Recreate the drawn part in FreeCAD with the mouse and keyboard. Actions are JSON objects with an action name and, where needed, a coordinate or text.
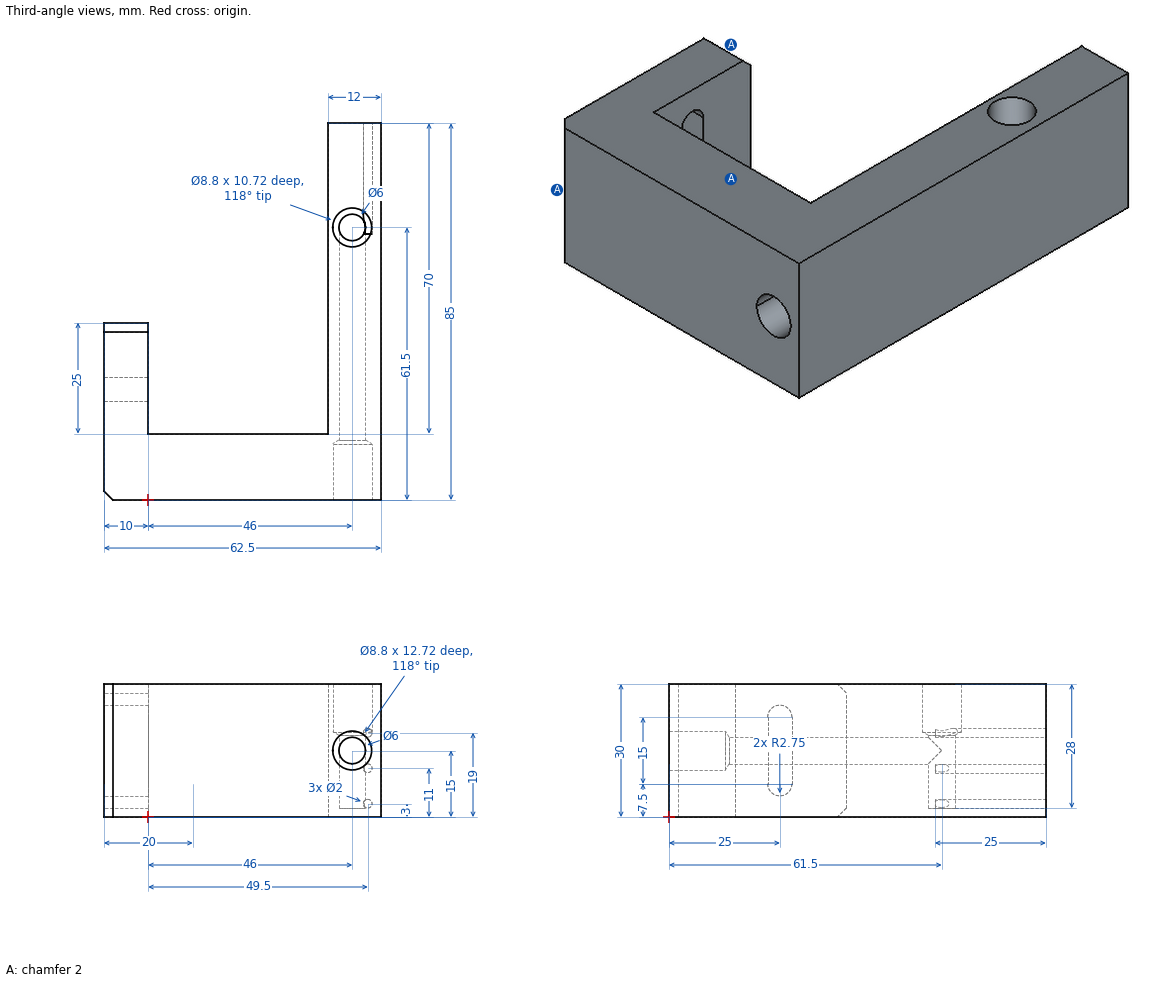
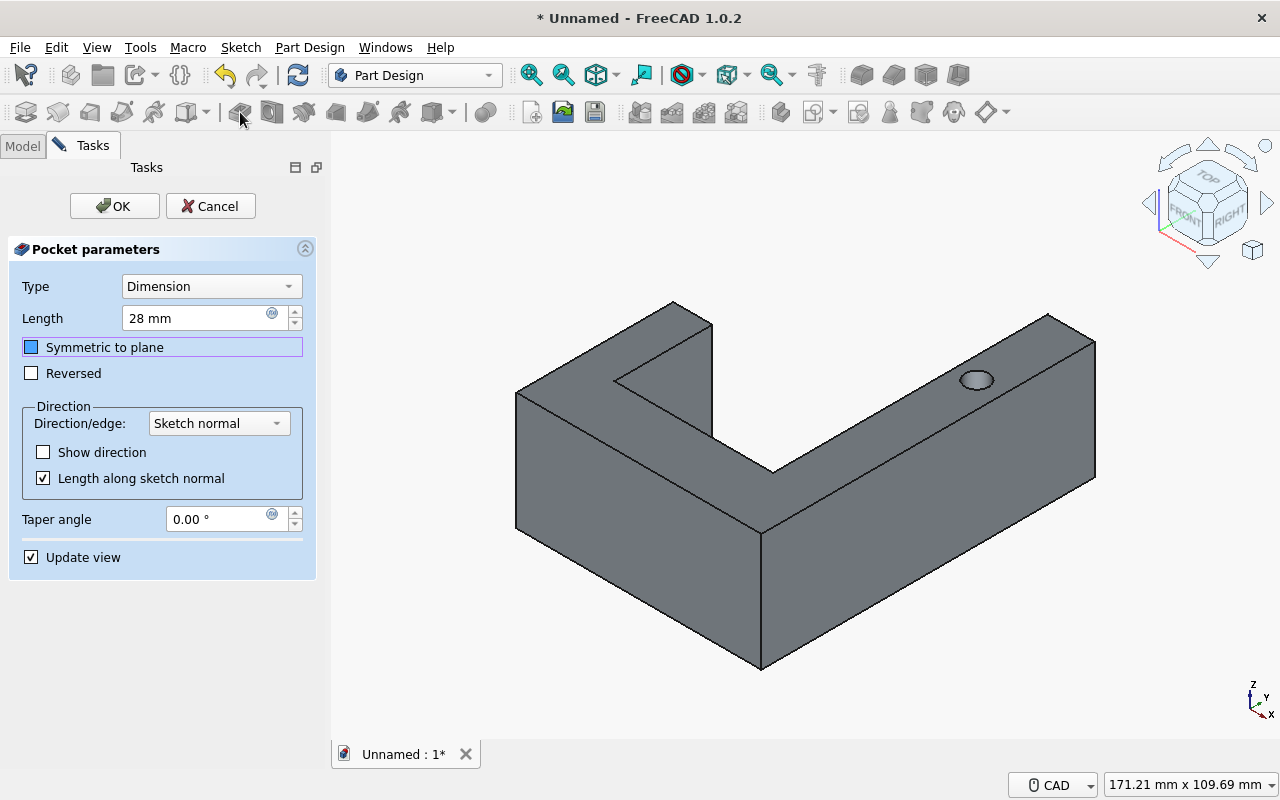
{"action": "left_click", "coordinate": [115, 206]}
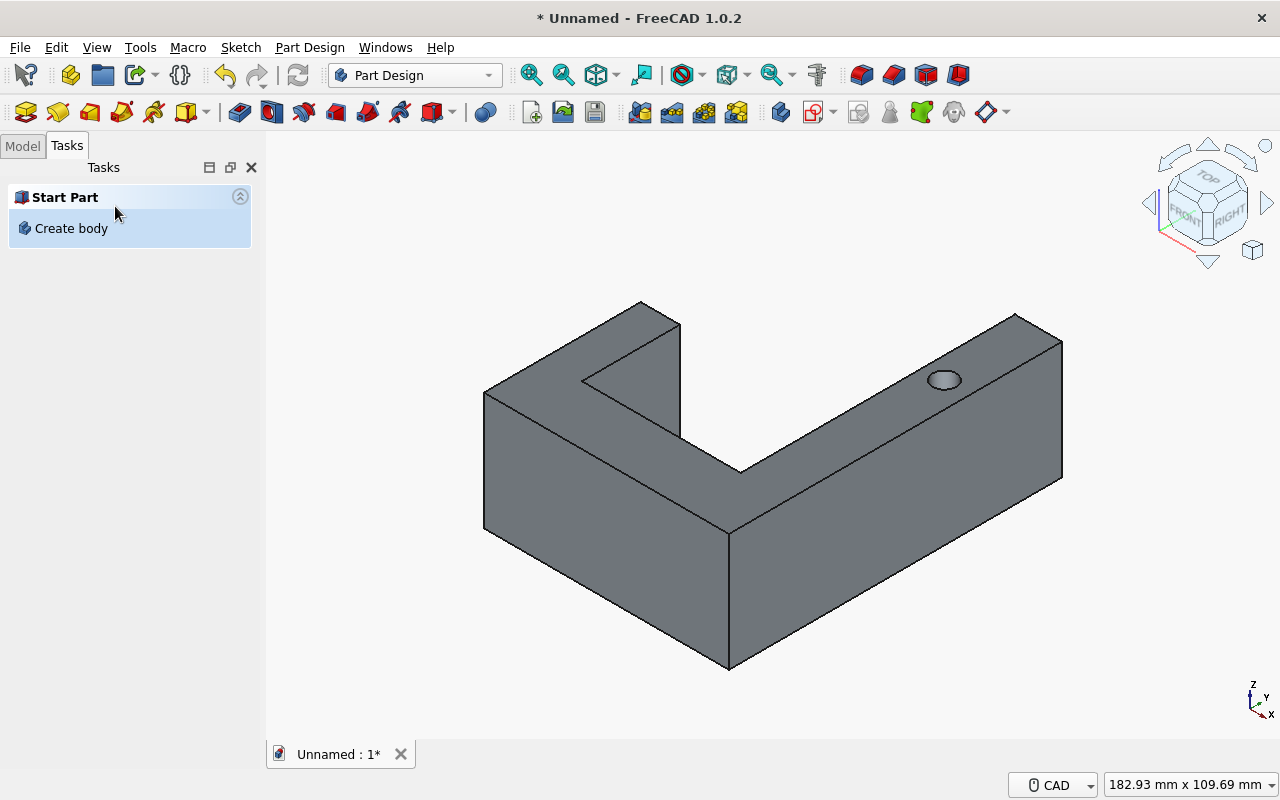
{"action": "left_click", "coordinate": [641, 550]}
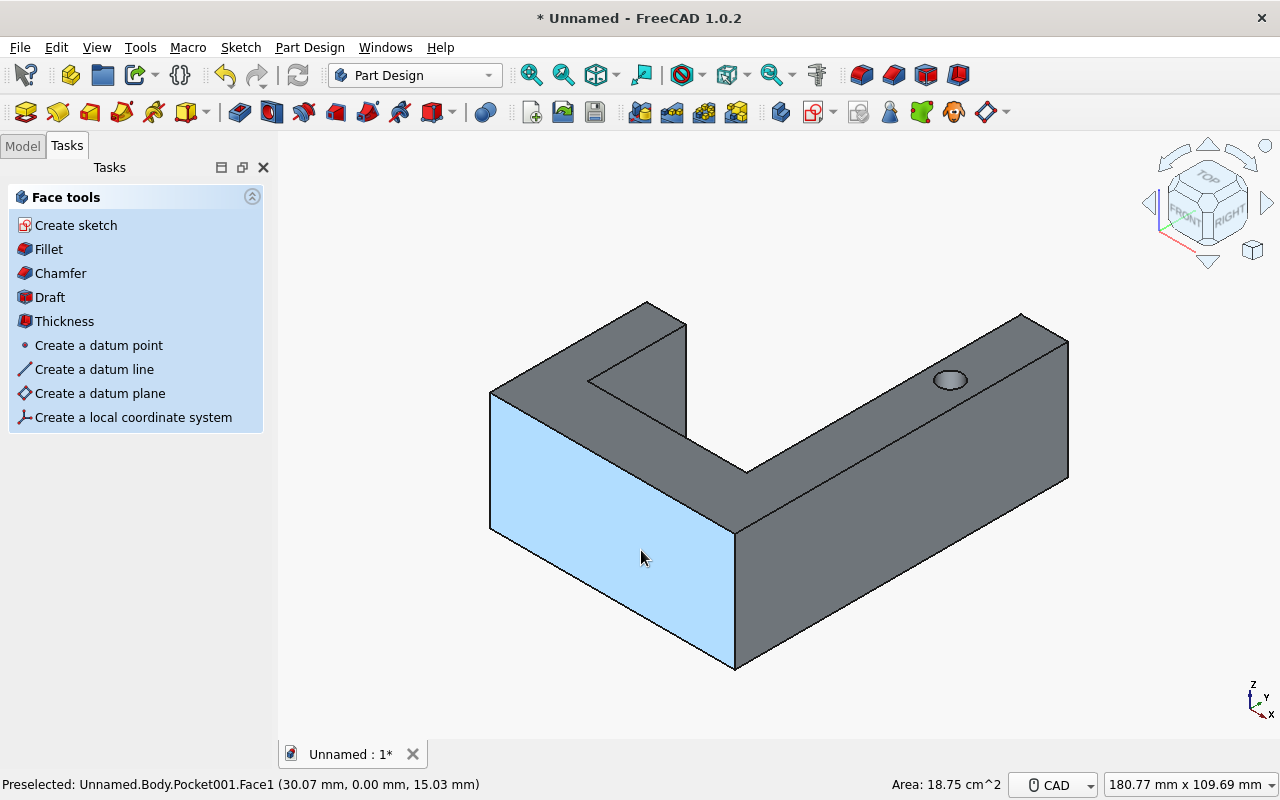
{"action": "left_click", "coordinate": [814, 112]}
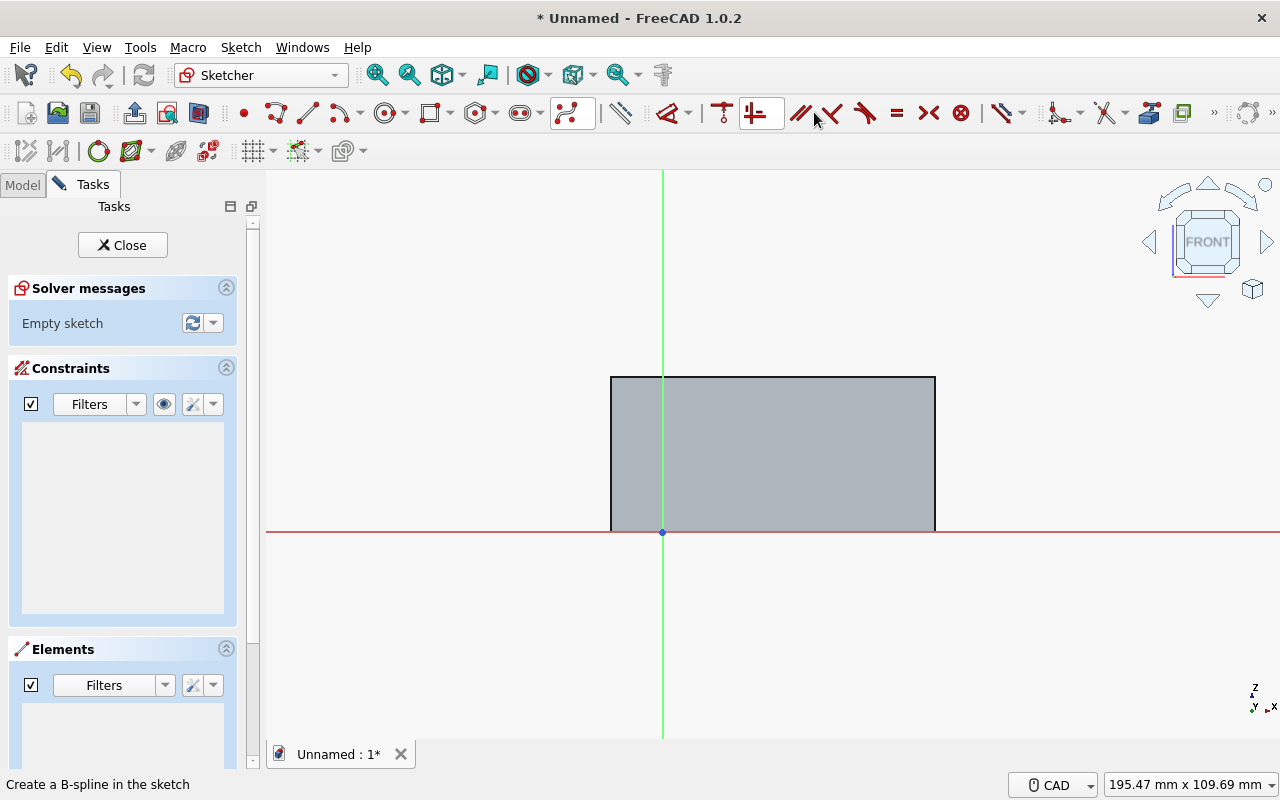
{"action": "scroll", "coordinate": [921, 455], "scroll_direction": "up", "scroll_amount": 12}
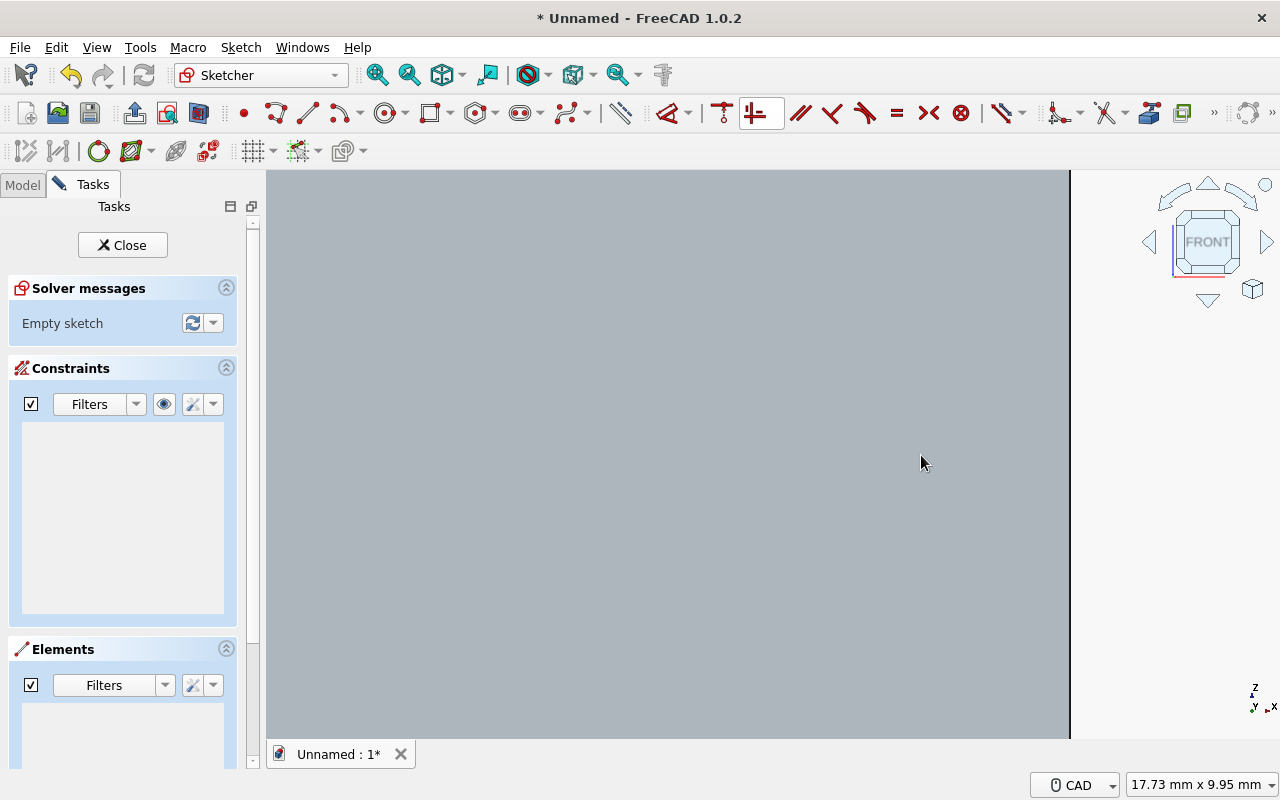
{"action": "key", "text": "g c"}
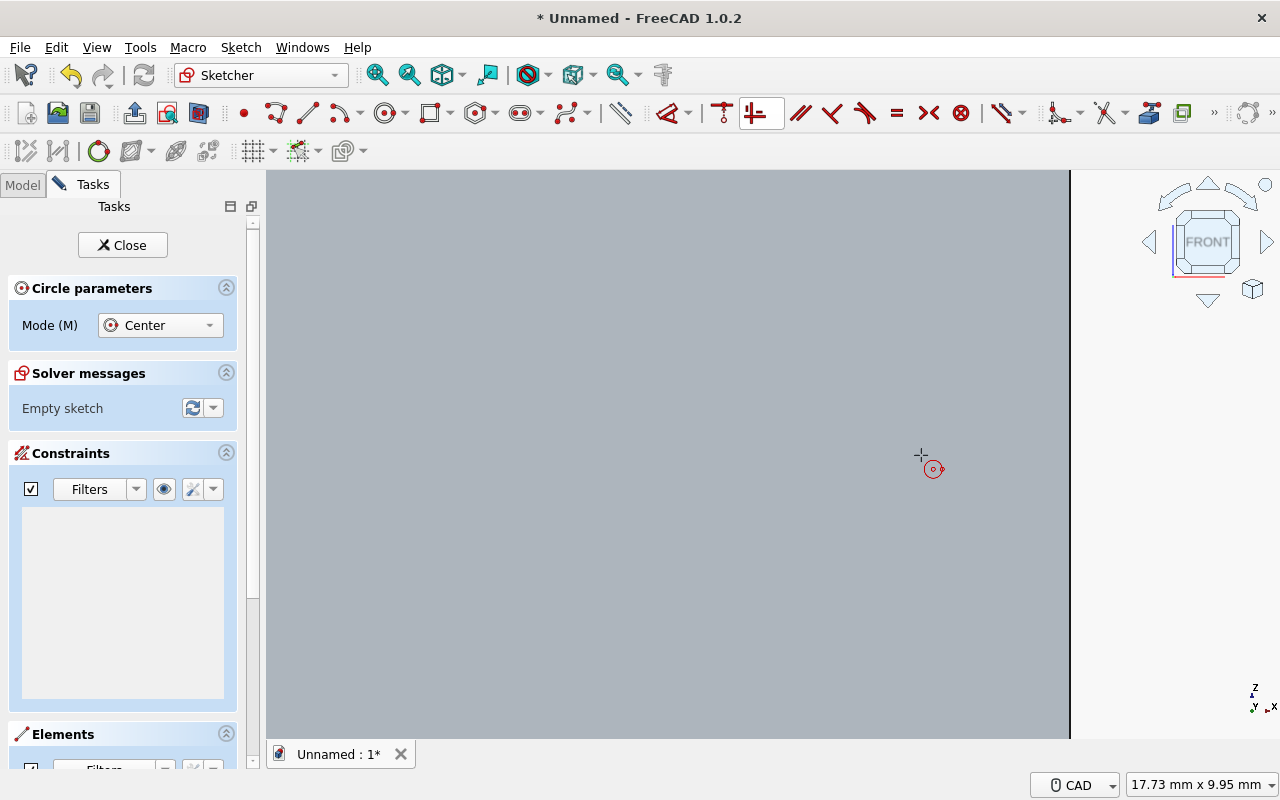
{"action": "left_click", "coordinate": [698, 444]}
{"action": "mouse_move", "coordinate": [820, 323]}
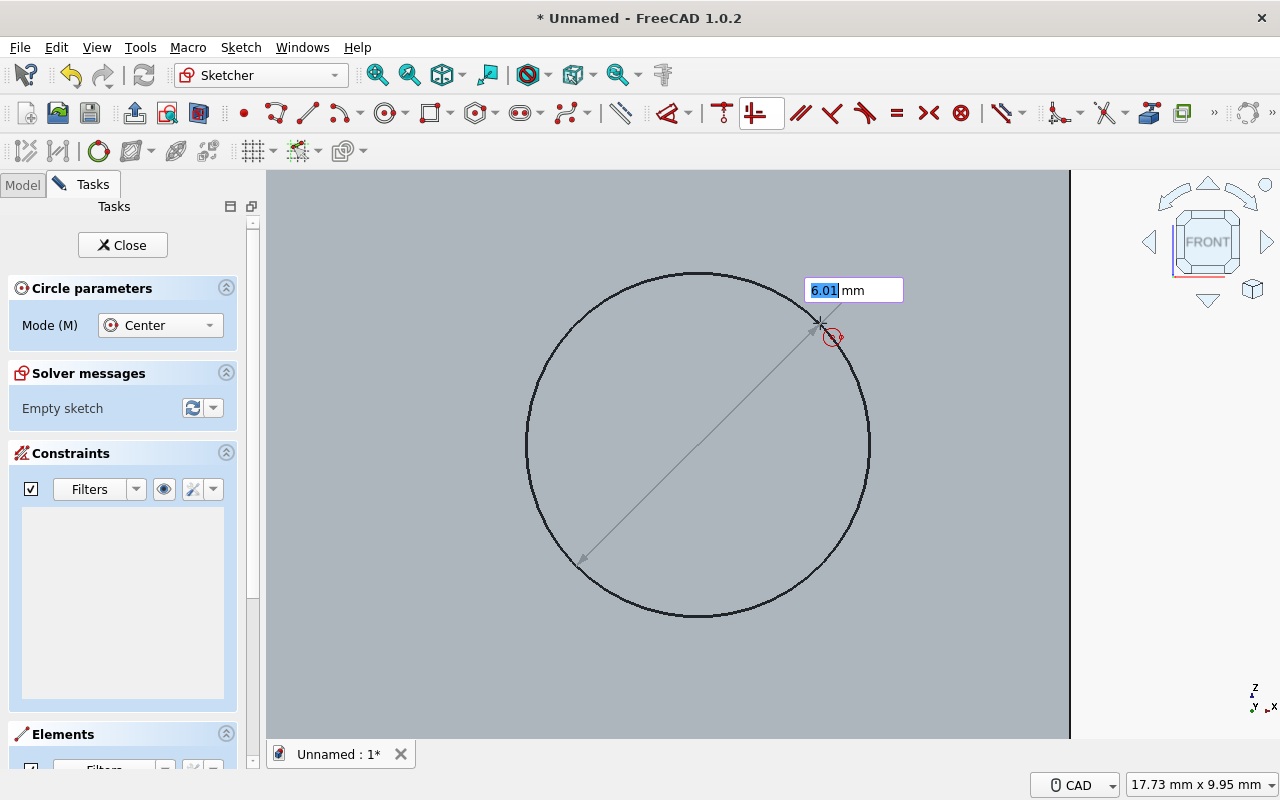
{"action": "type", "text": "6"}
{"action": "key", "text": "Return"}
{"action": "key", "text": "Escape"}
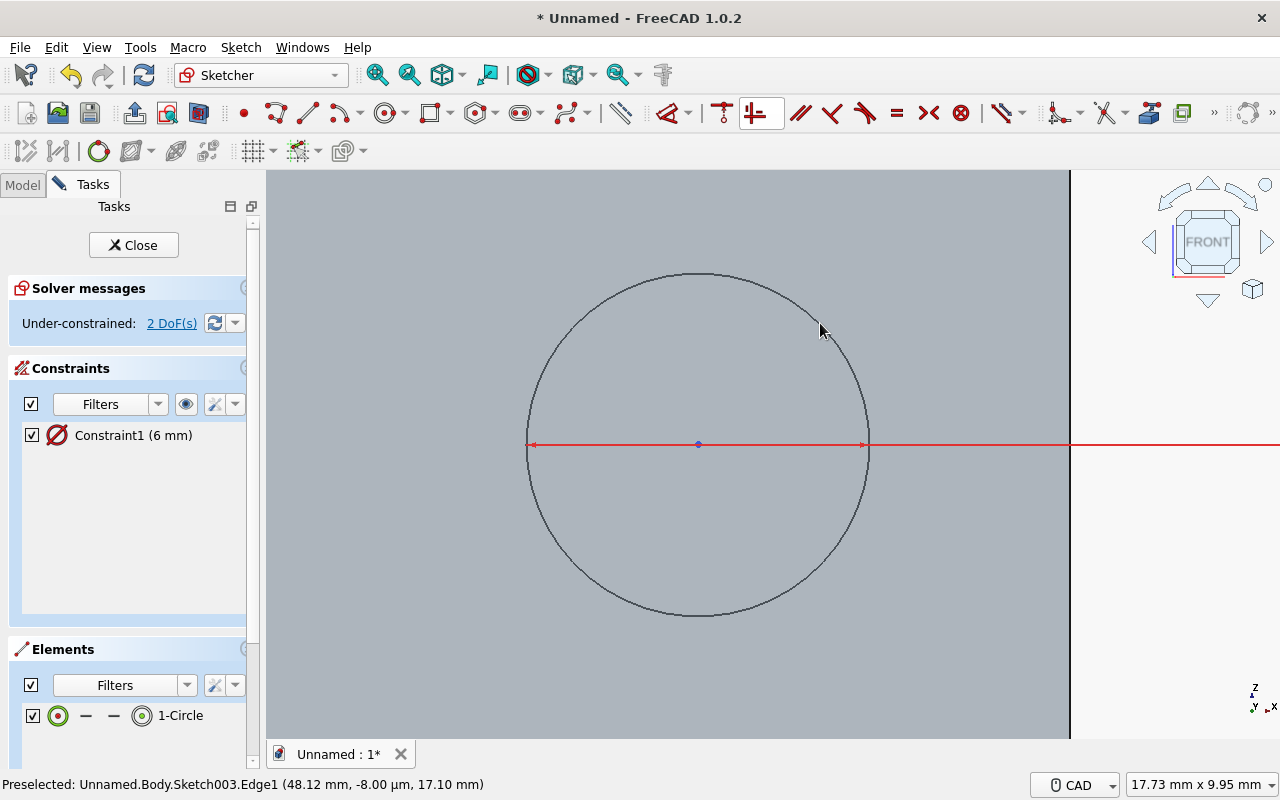
{"action": "key", "text": "d"}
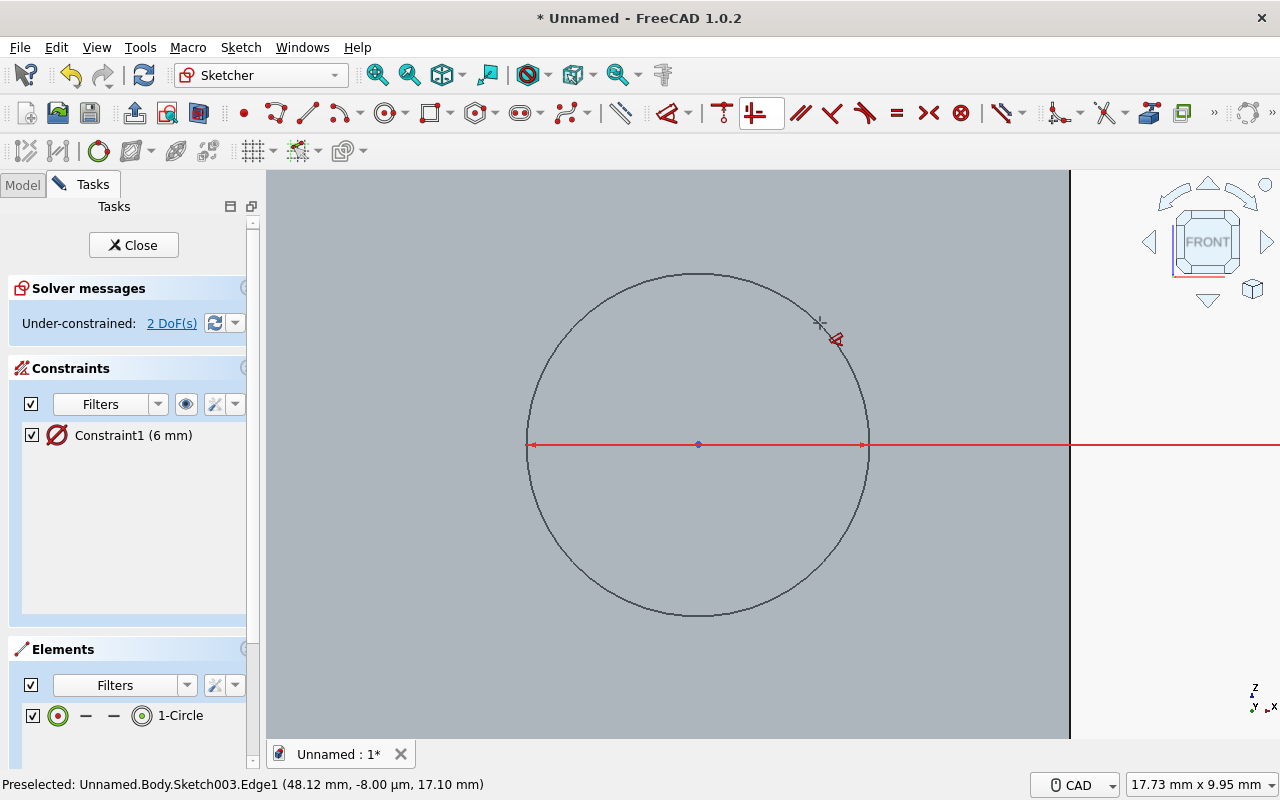
{"action": "left_click", "coordinate": [698, 445]}
{"action": "left_click", "coordinate": [496, 411]}